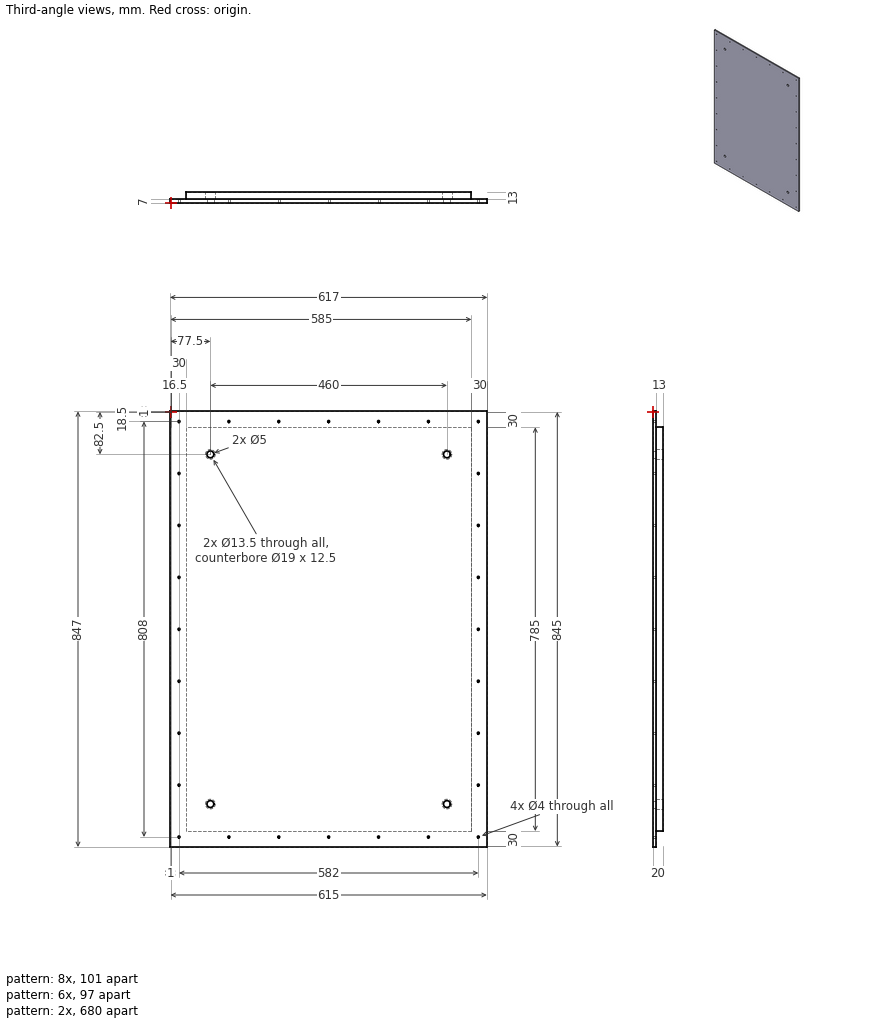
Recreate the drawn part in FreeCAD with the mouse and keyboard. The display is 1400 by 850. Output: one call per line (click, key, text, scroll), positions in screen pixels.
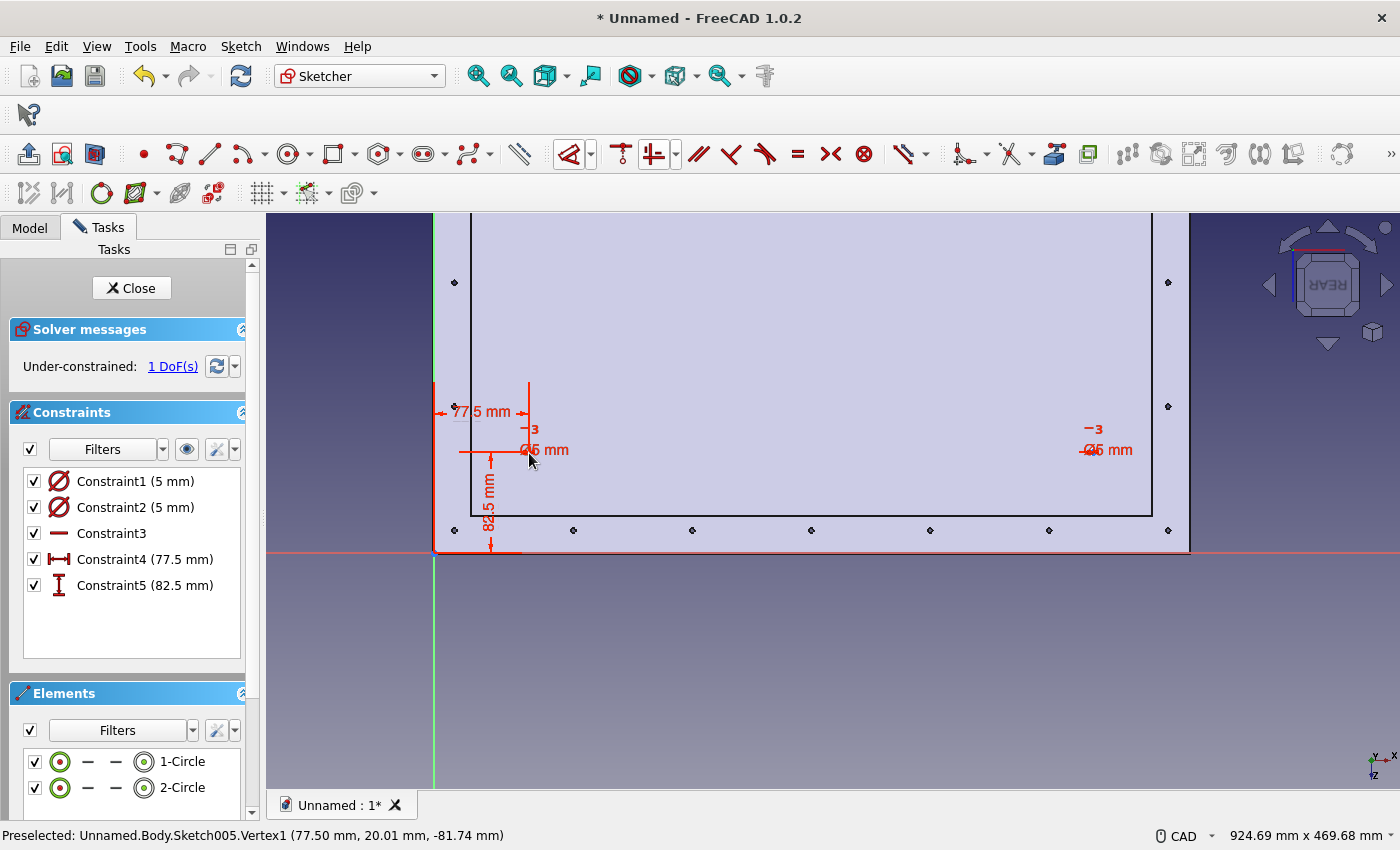
click(529, 452)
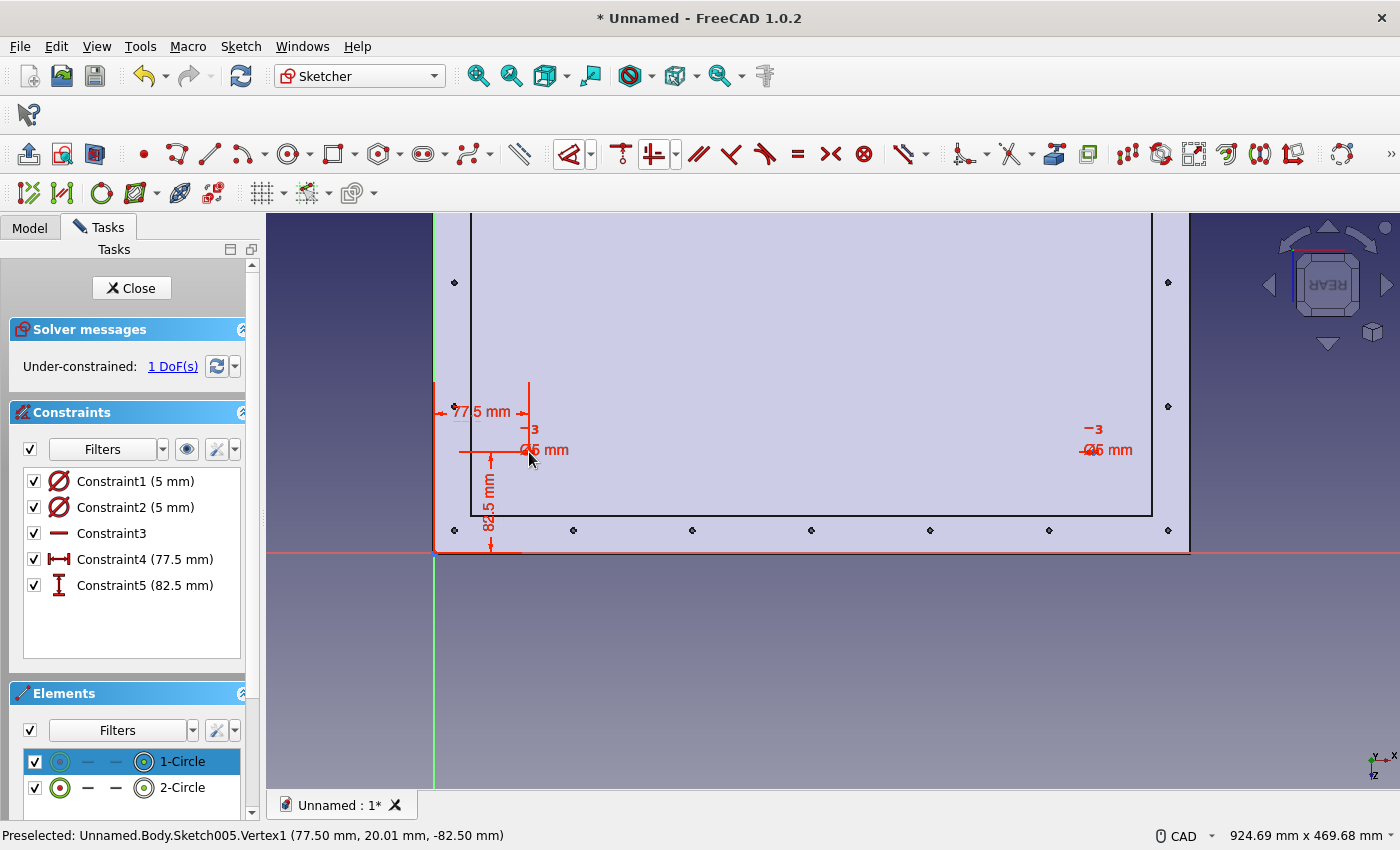
click(1093, 452)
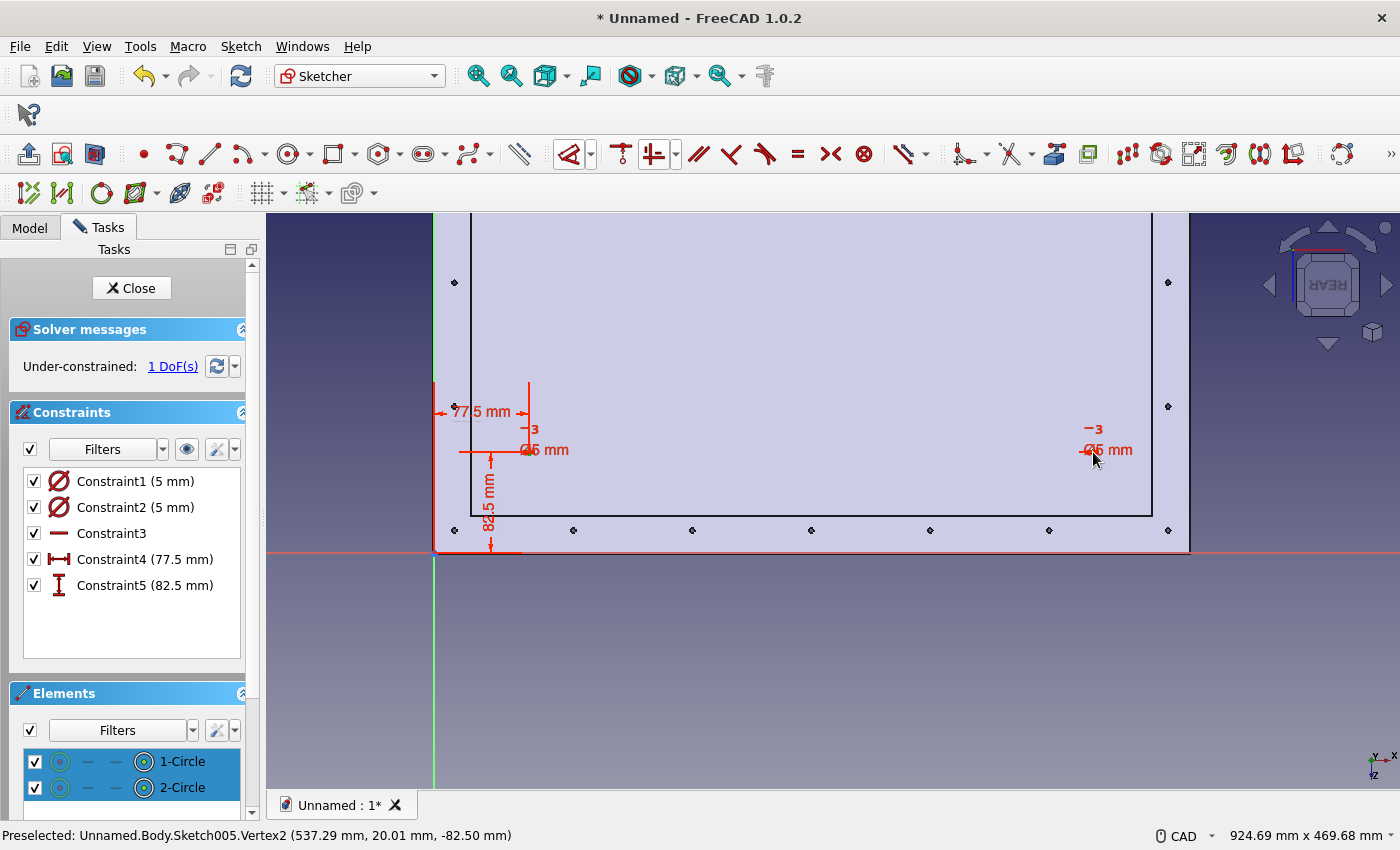
click(590, 154)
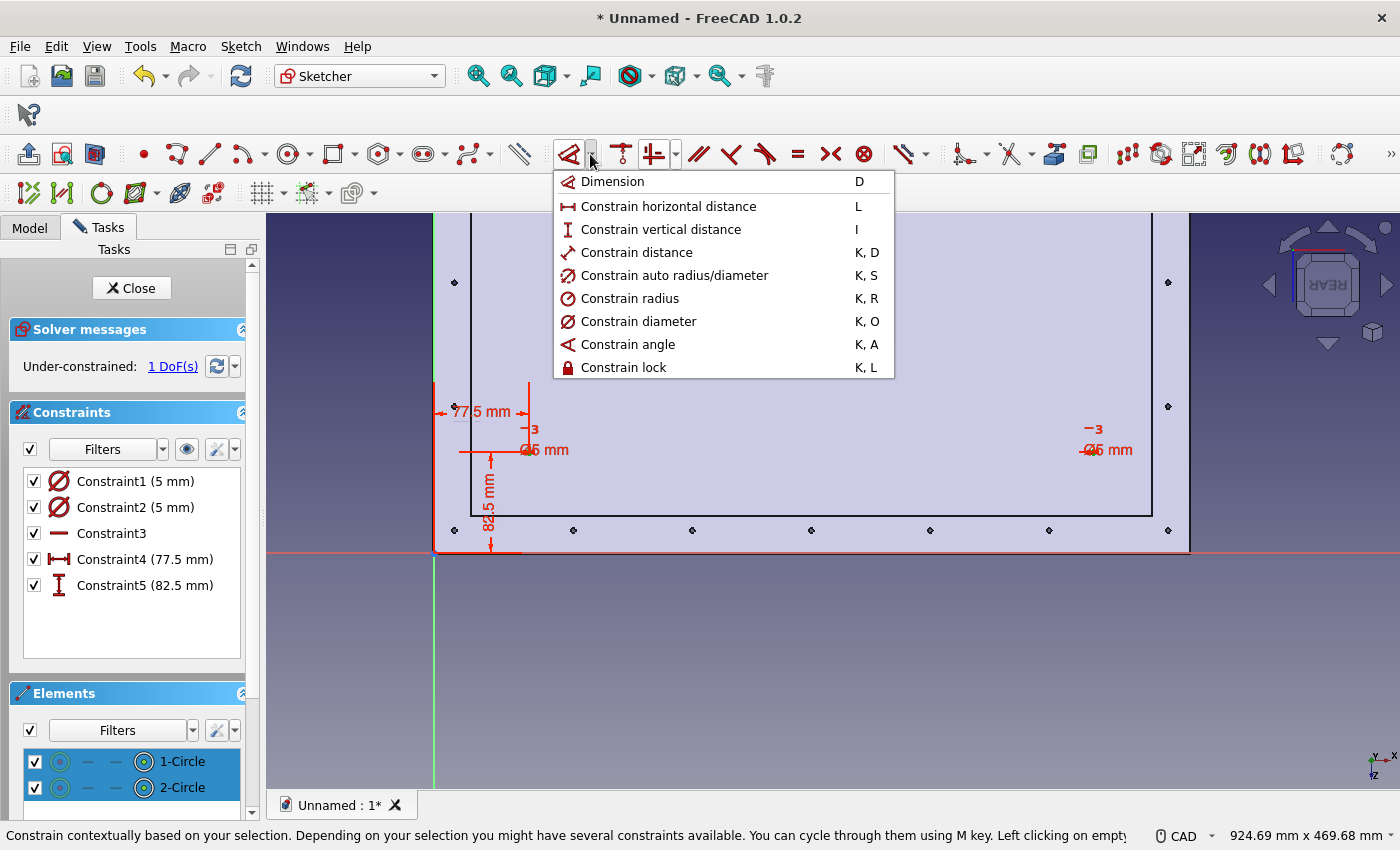
click(724, 206)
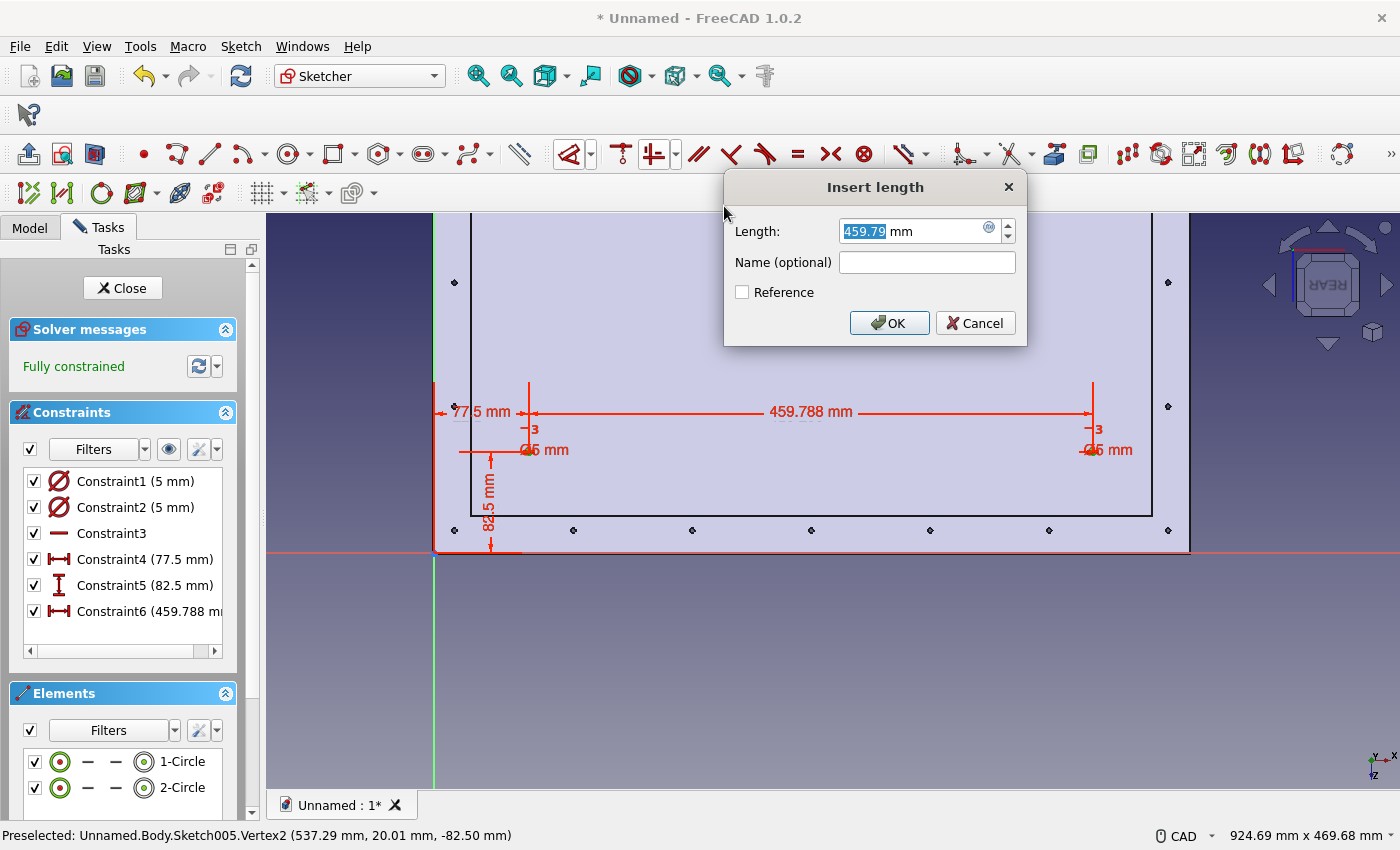
text(460)
key(Return)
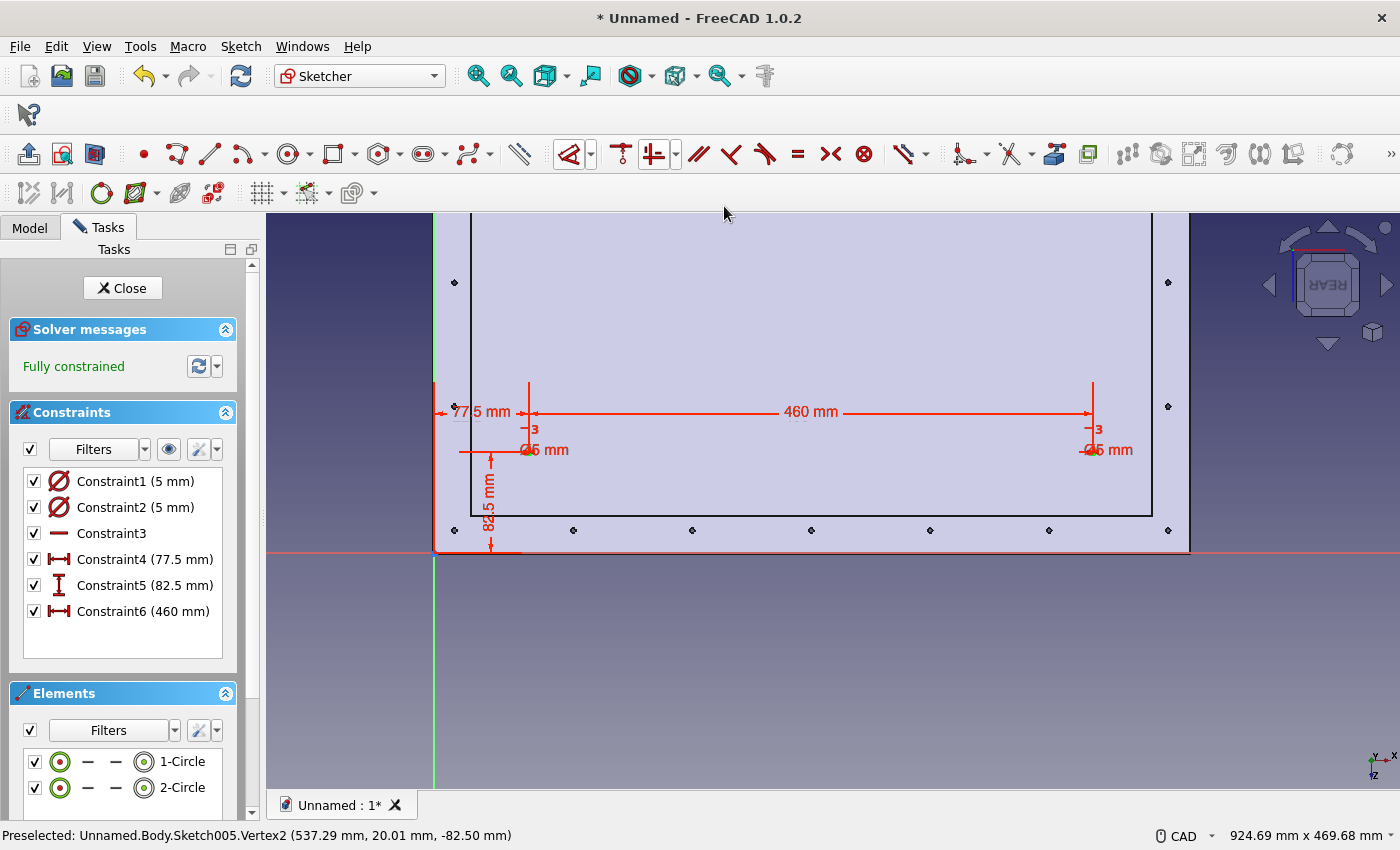
click(123, 288)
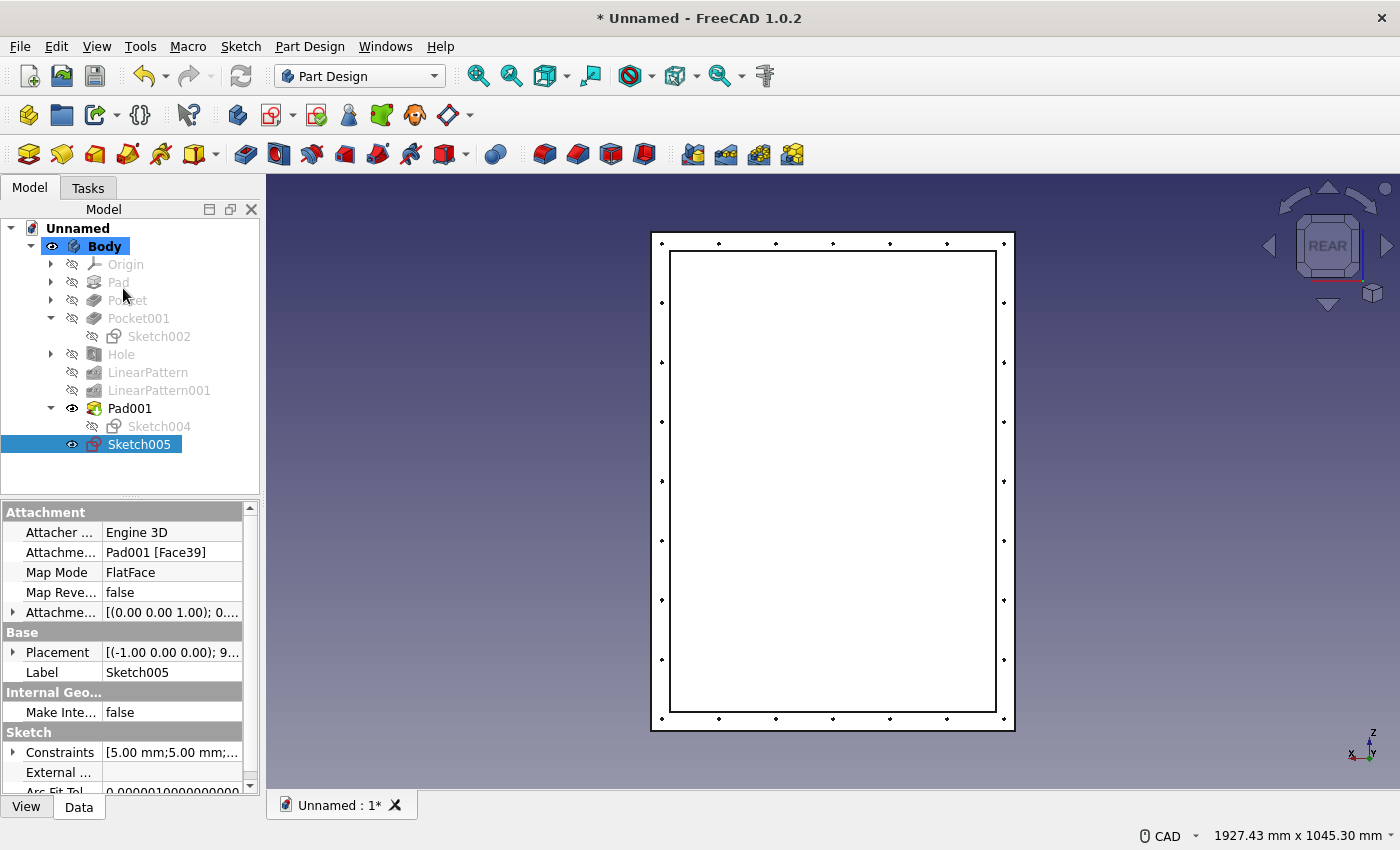
click(246, 154)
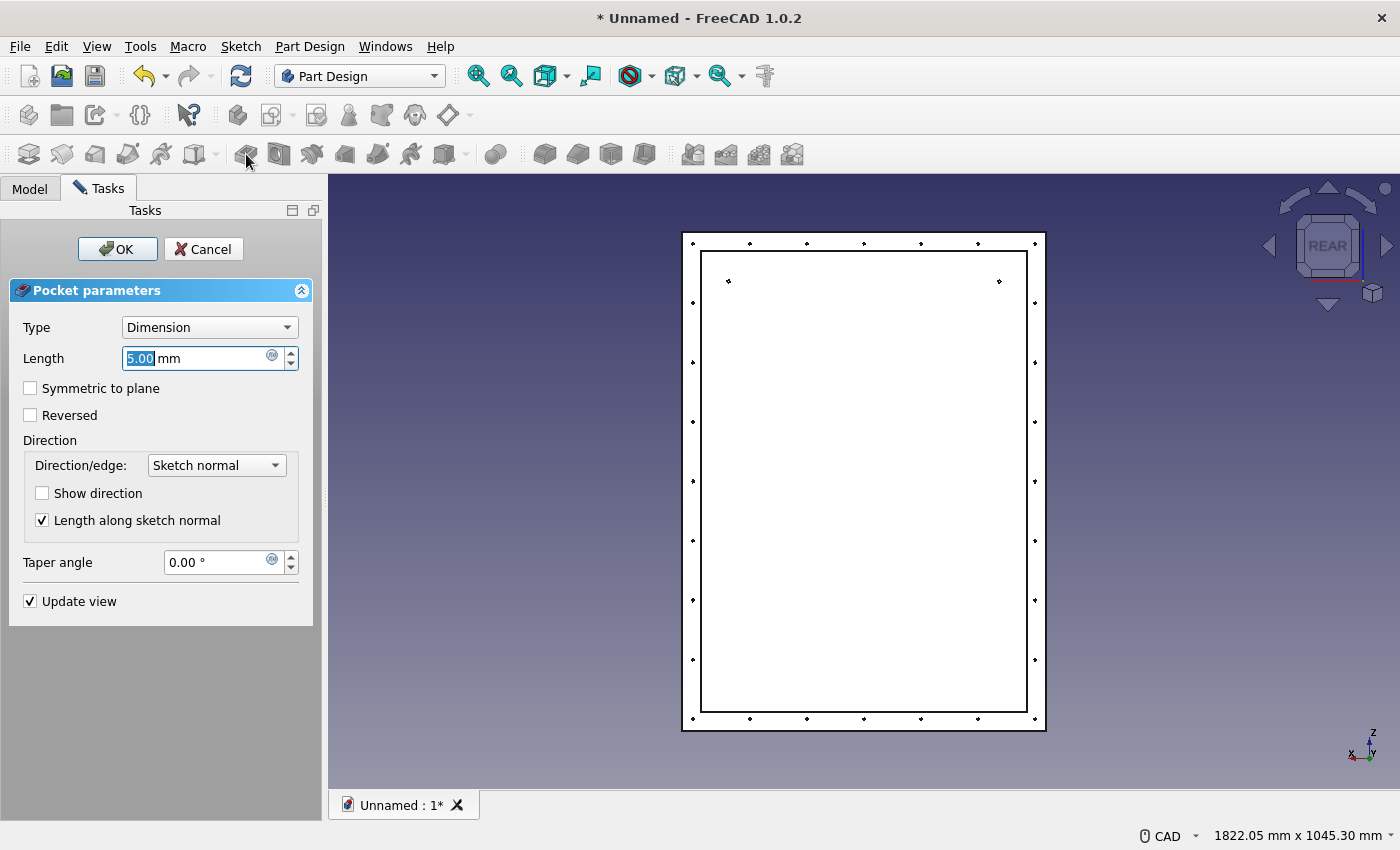
text(20)
key(Tab)